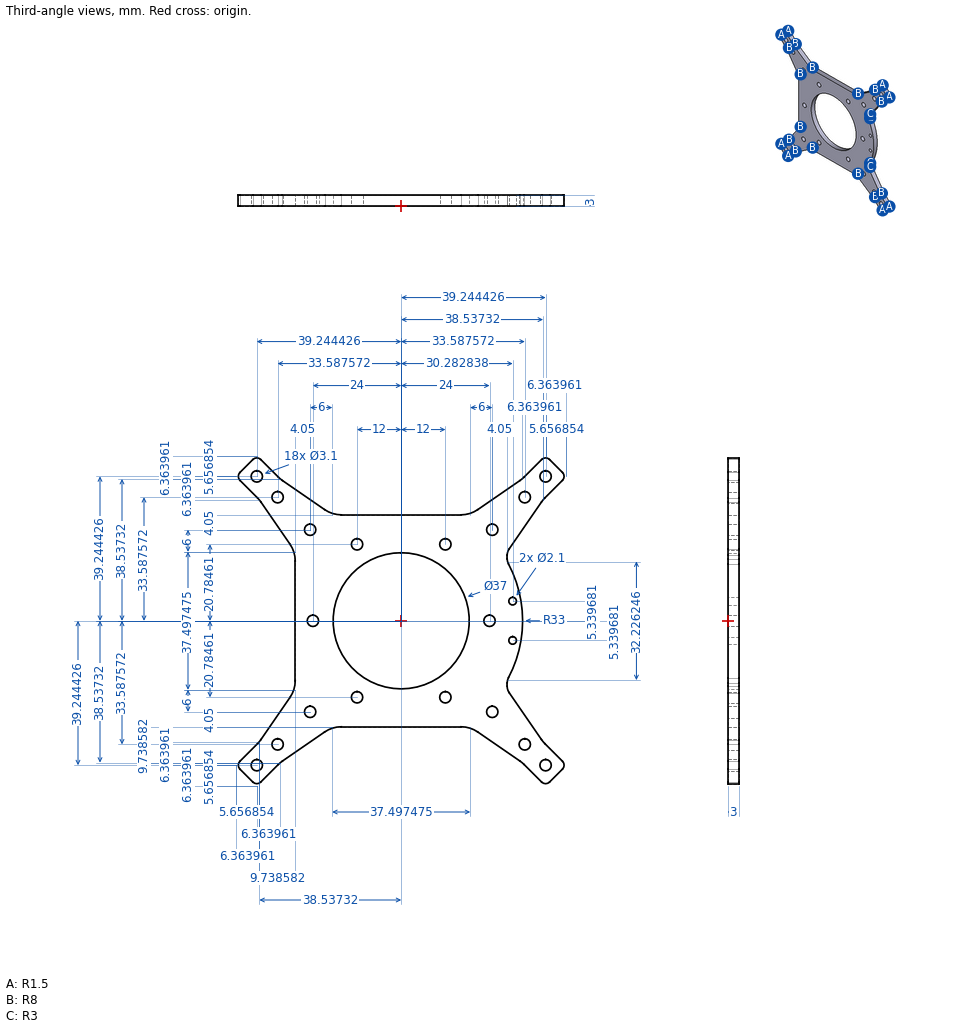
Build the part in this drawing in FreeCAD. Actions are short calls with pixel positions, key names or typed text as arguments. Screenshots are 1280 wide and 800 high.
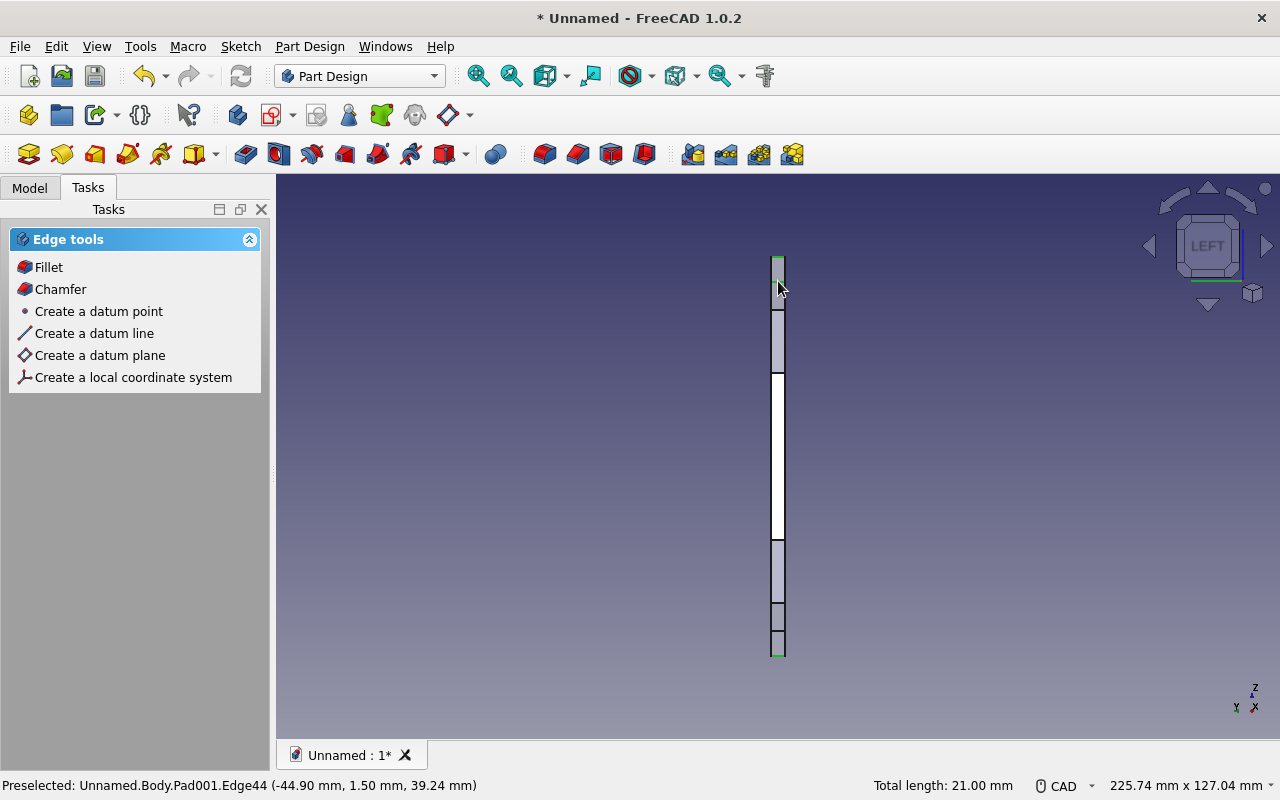
click(778, 630, ctrl)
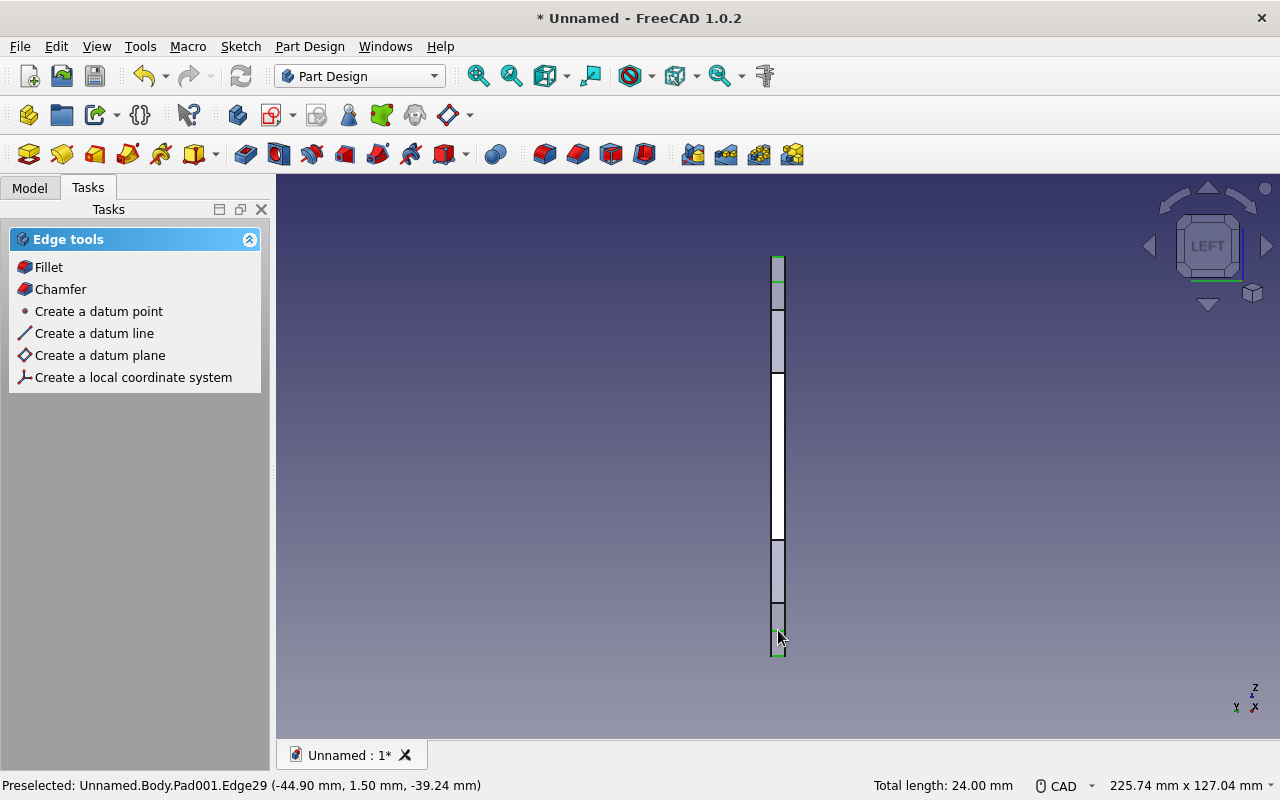
click(545, 154)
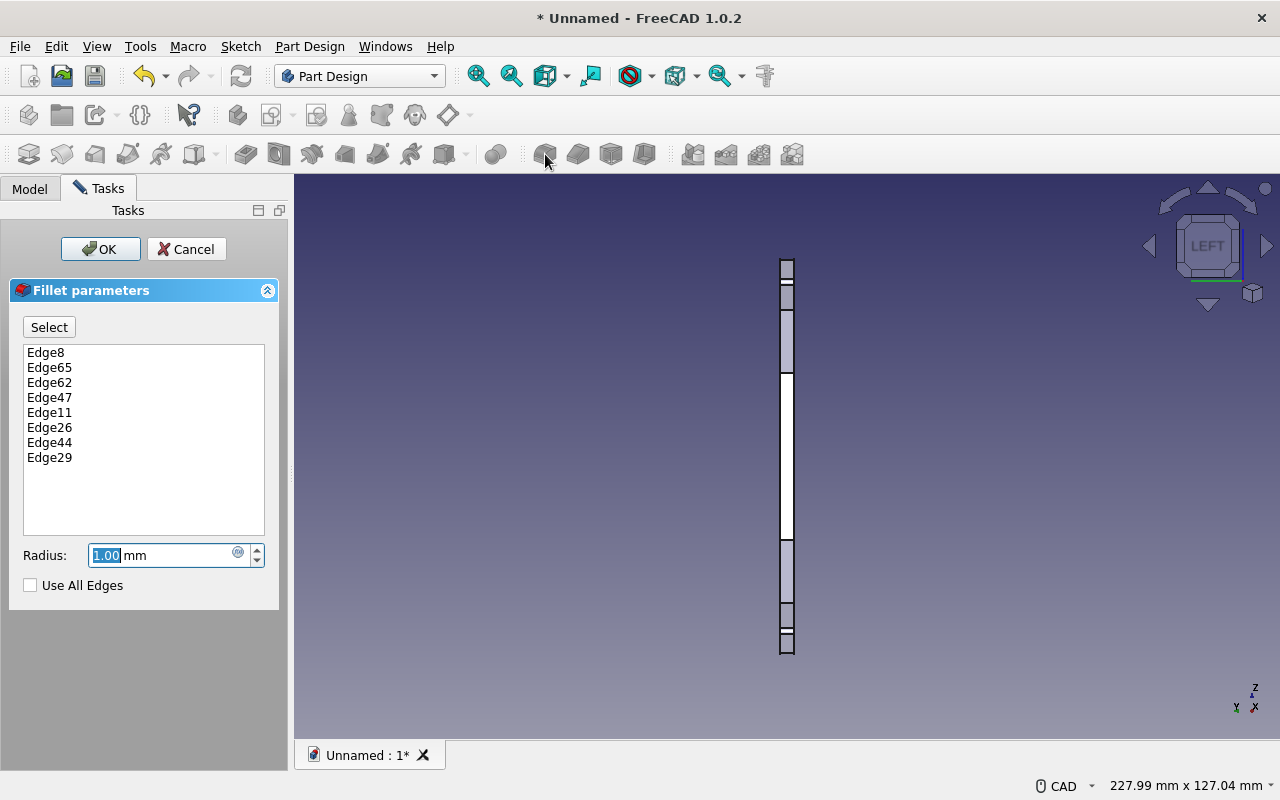
text(1.5)
key(Tab)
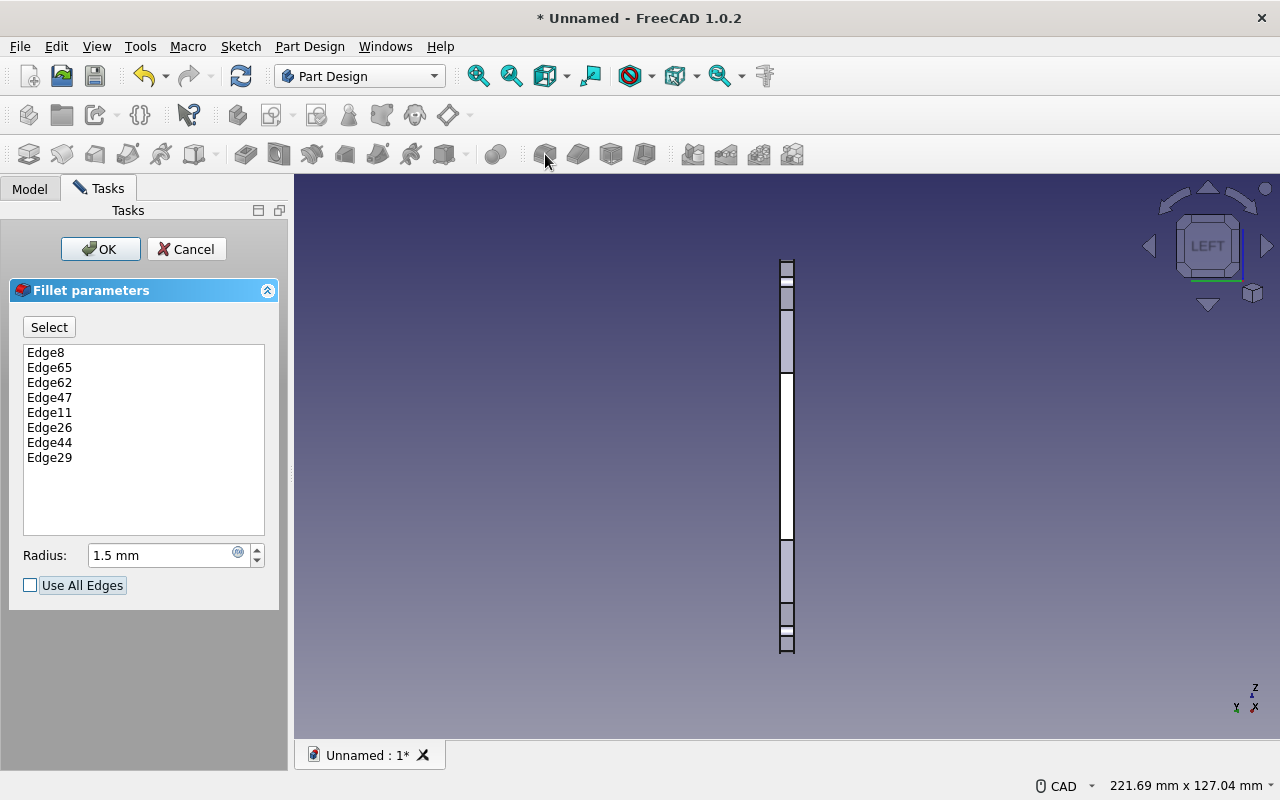
click(101, 249)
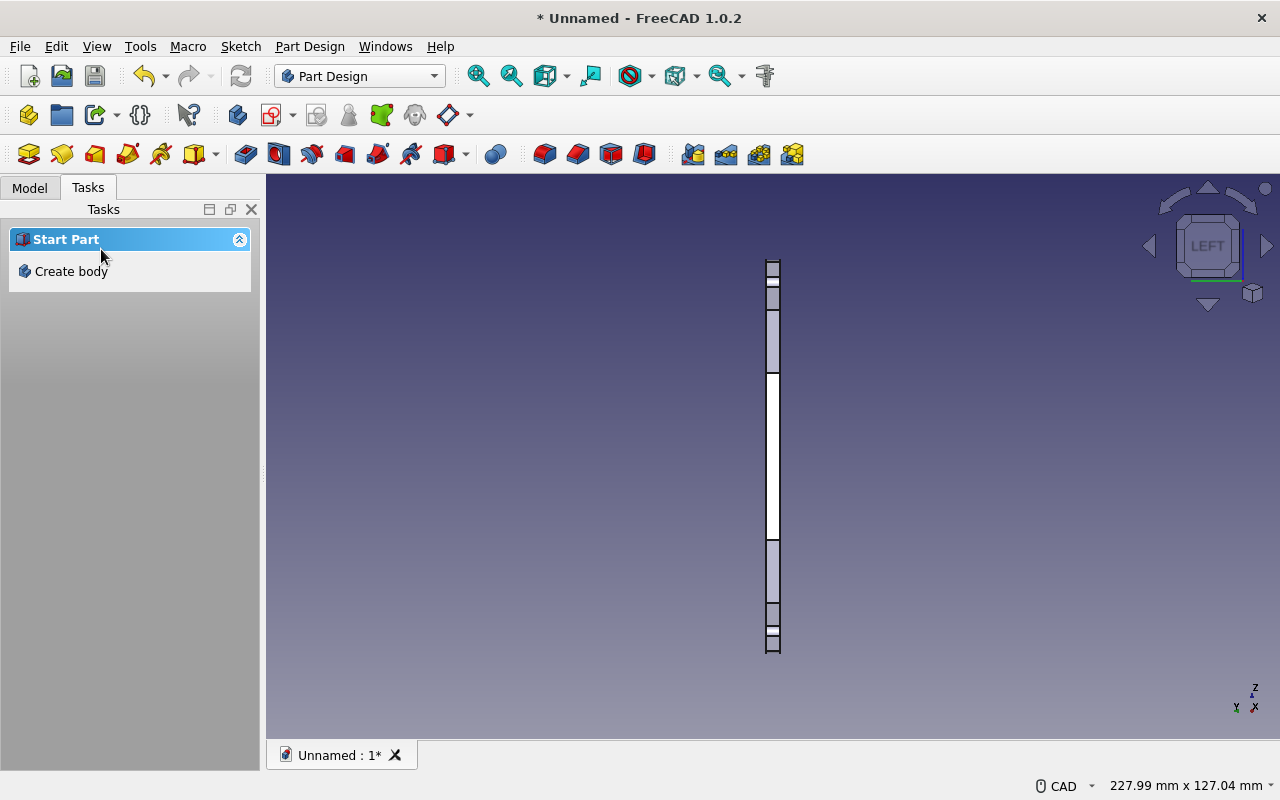
scroll(773, 584, up, 6)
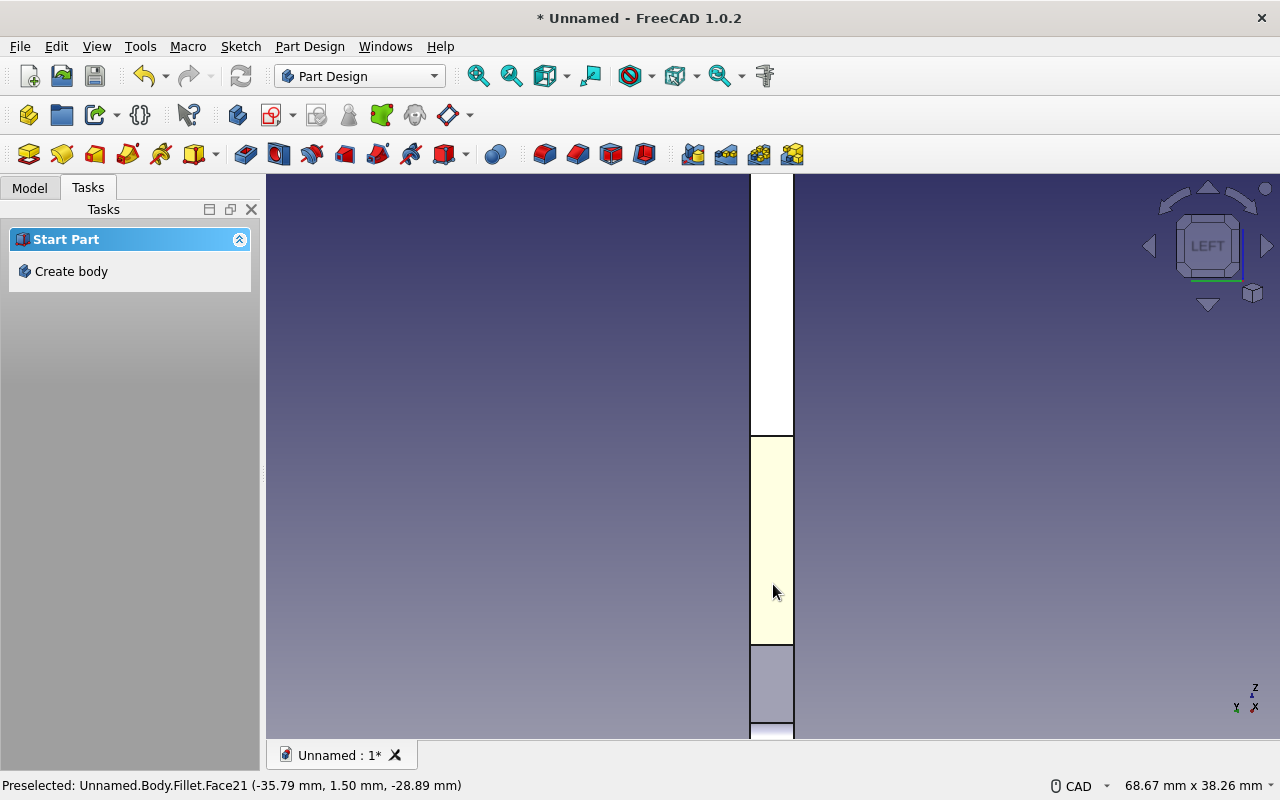
click(479, 76)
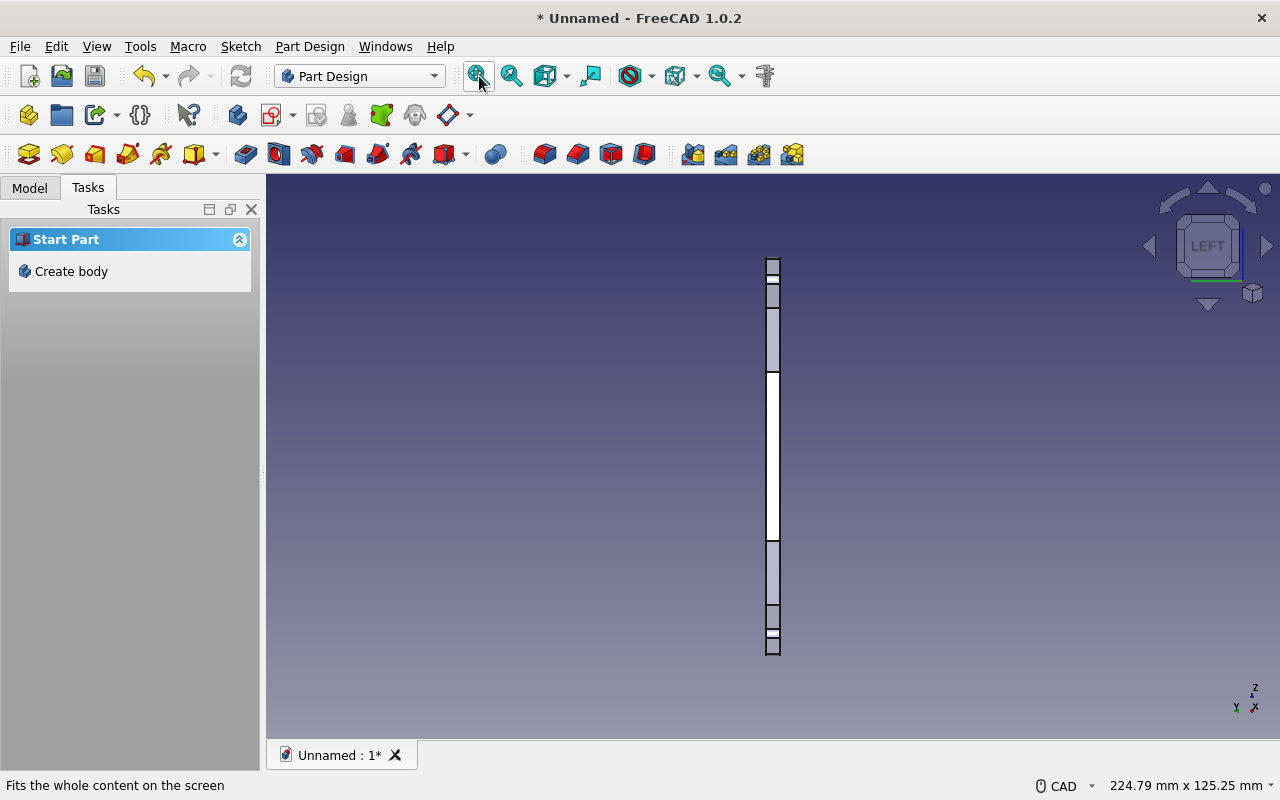
key(0)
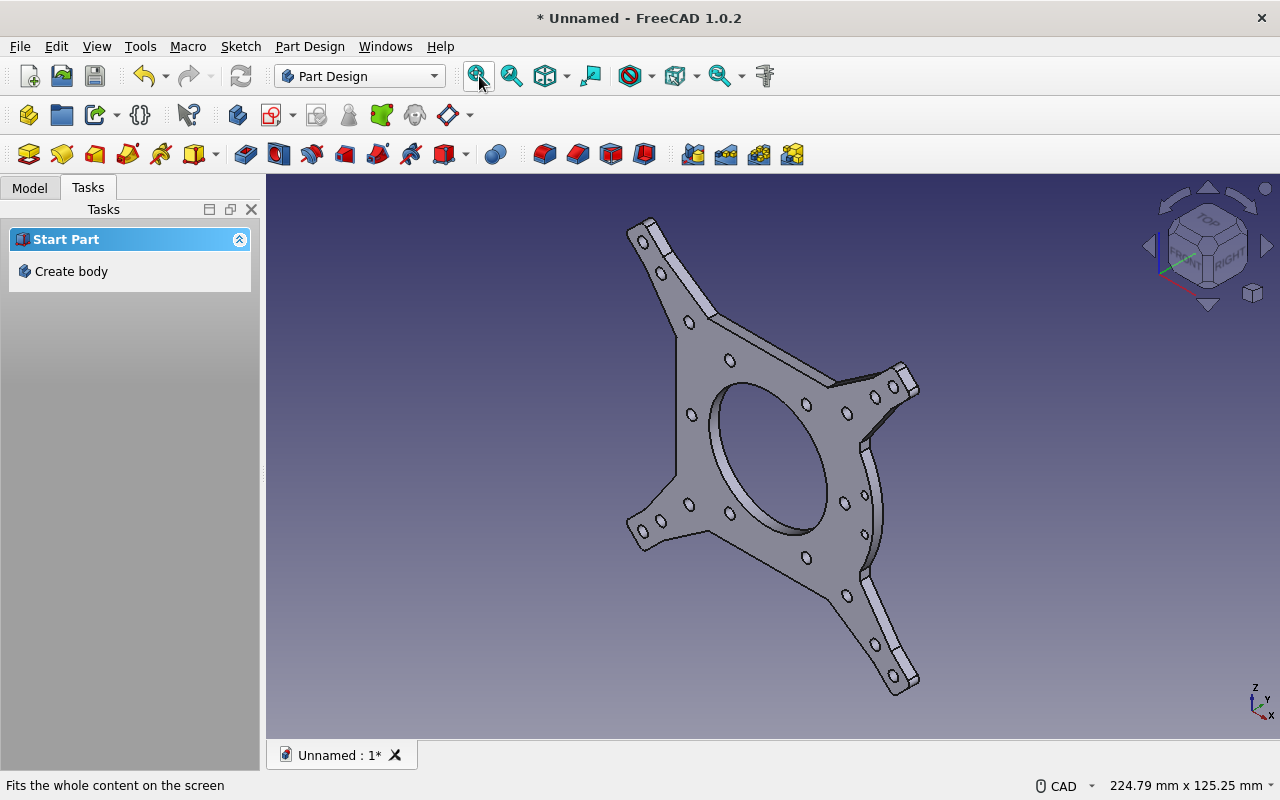
scroll(833, 596, up, 6)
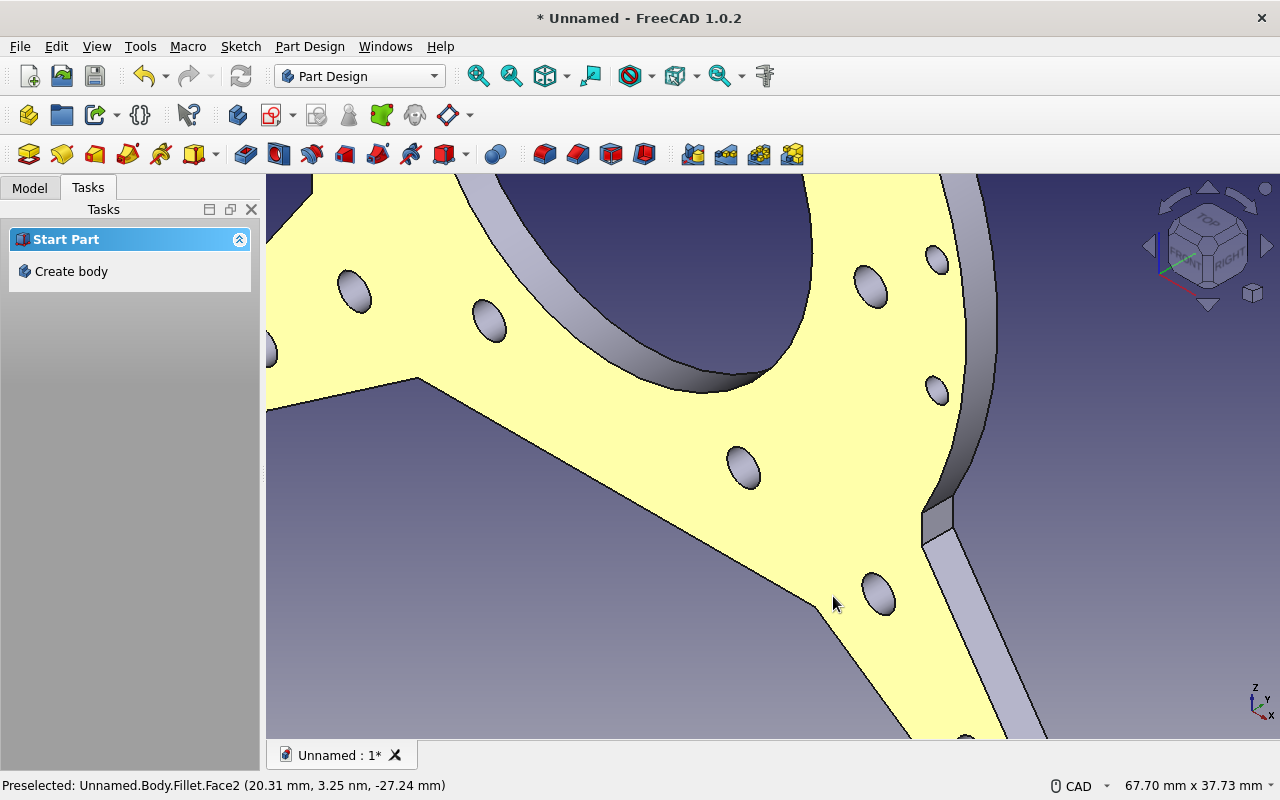
click(479, 76)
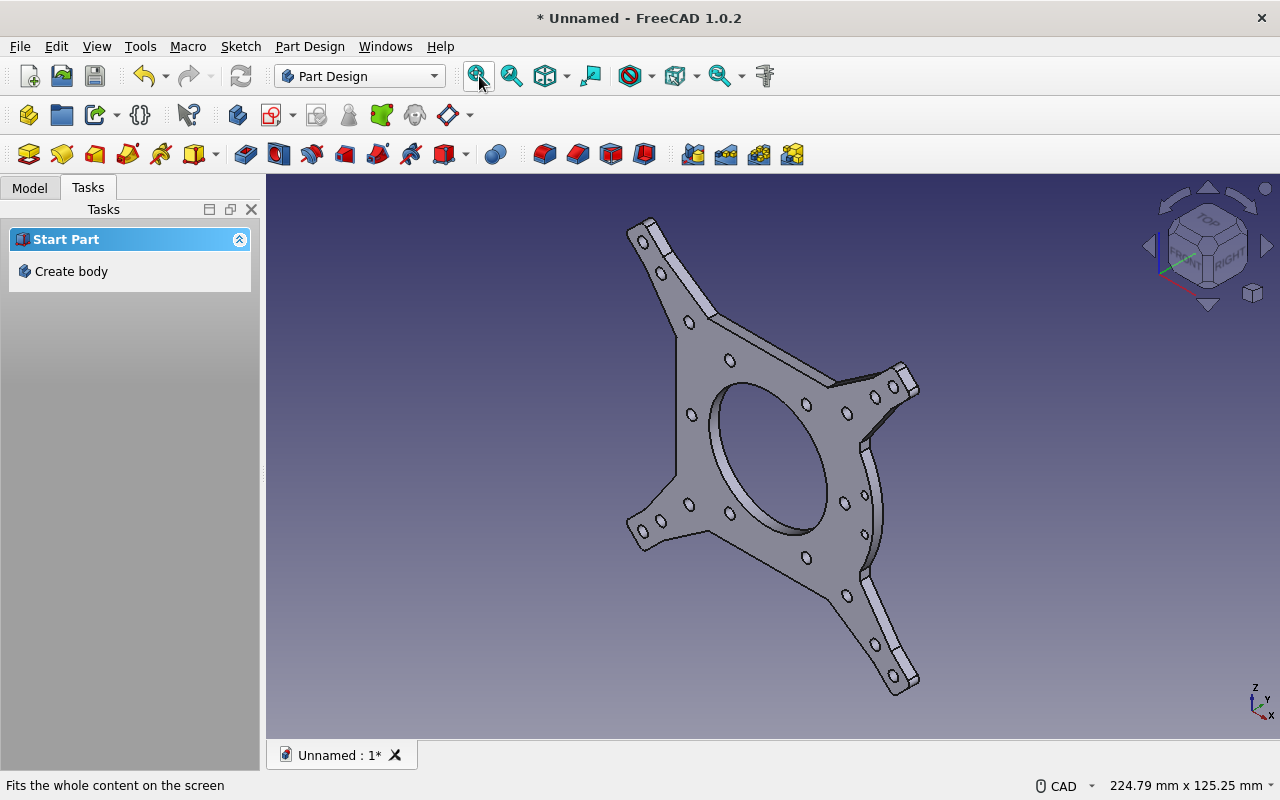
key(2)